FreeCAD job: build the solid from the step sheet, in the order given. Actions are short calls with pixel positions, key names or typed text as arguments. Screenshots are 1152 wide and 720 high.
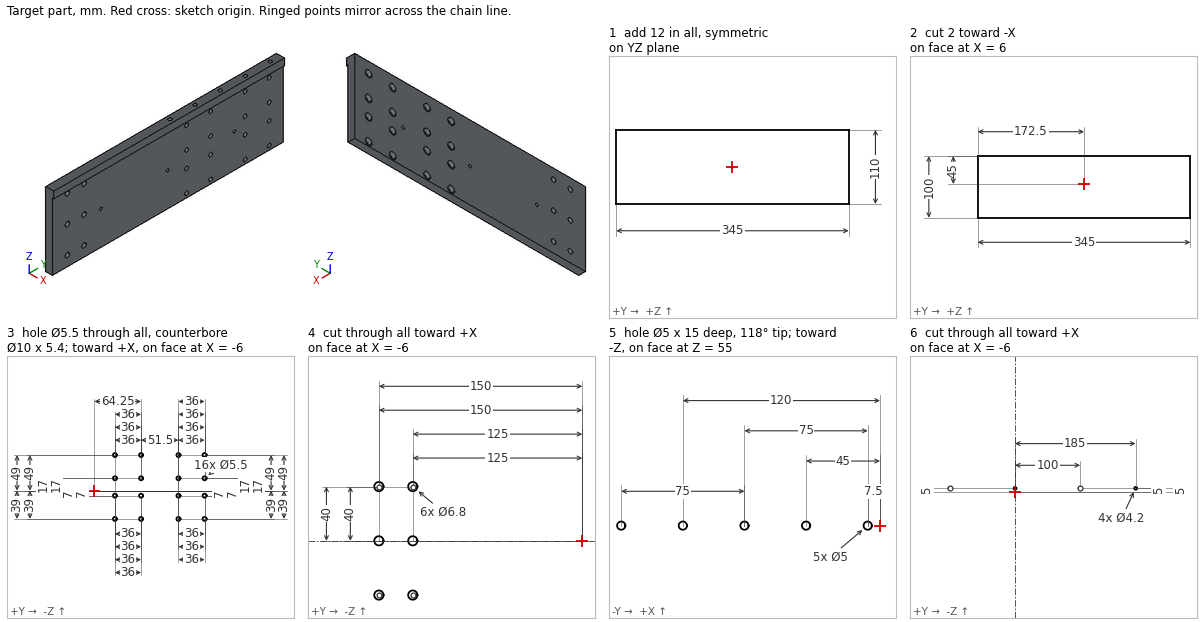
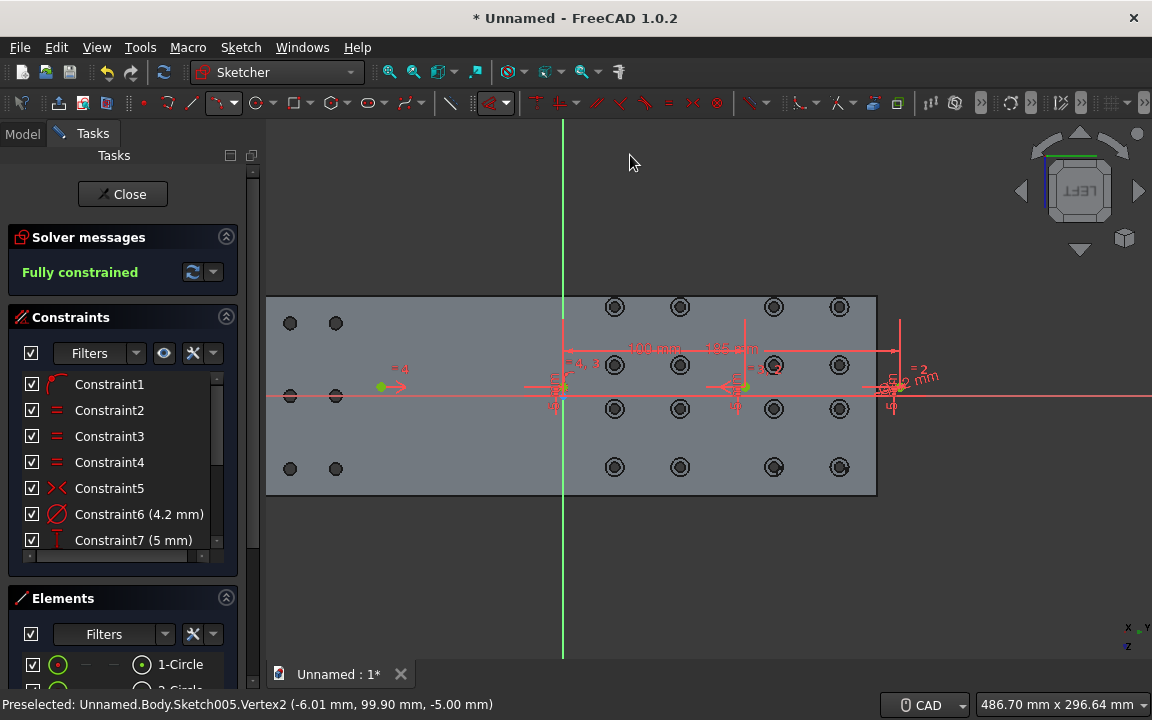
click(123, 194)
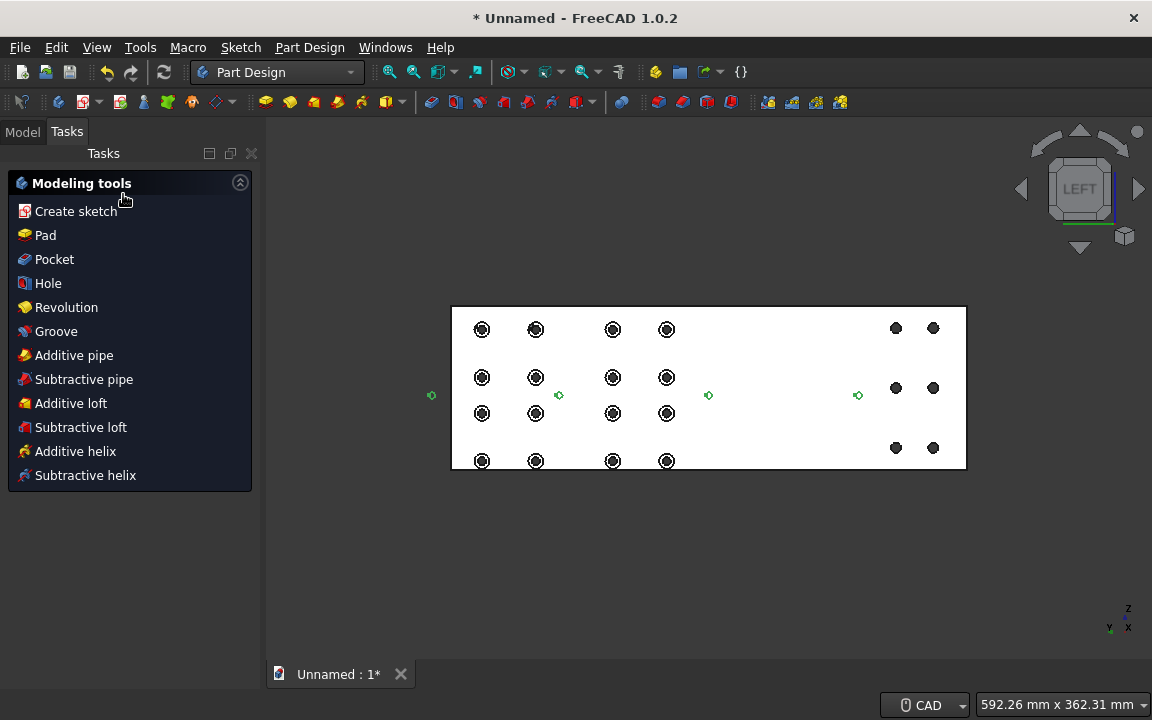
click(432, 102)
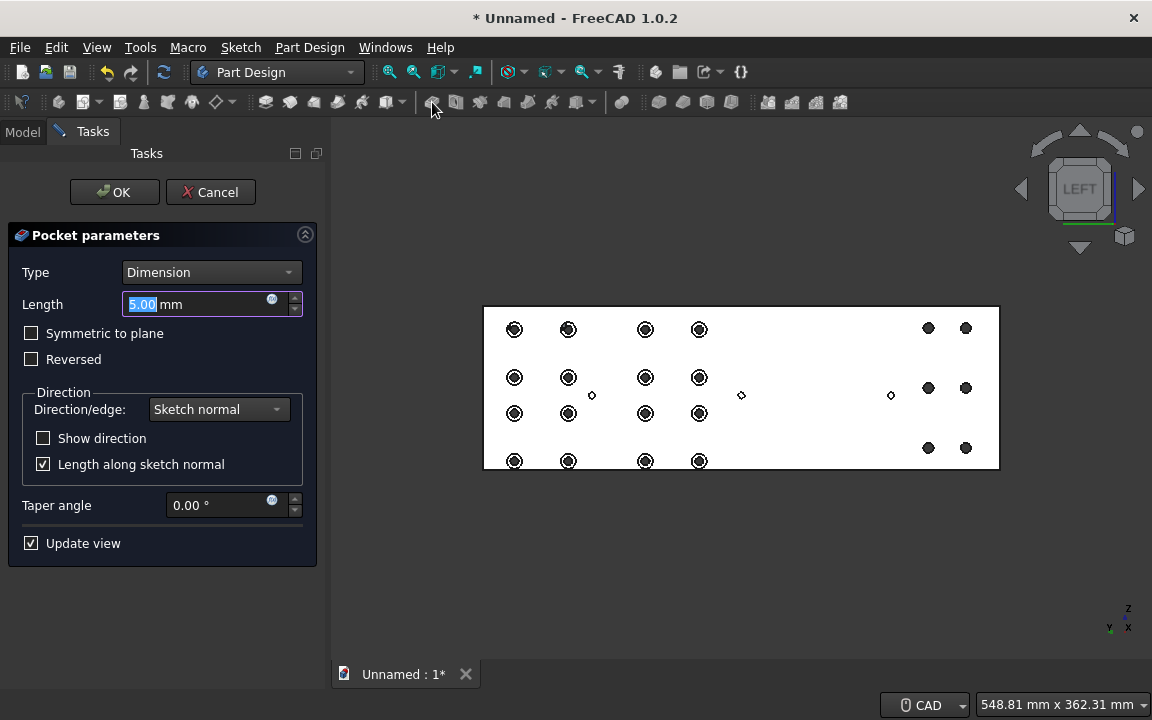
click(212, 272)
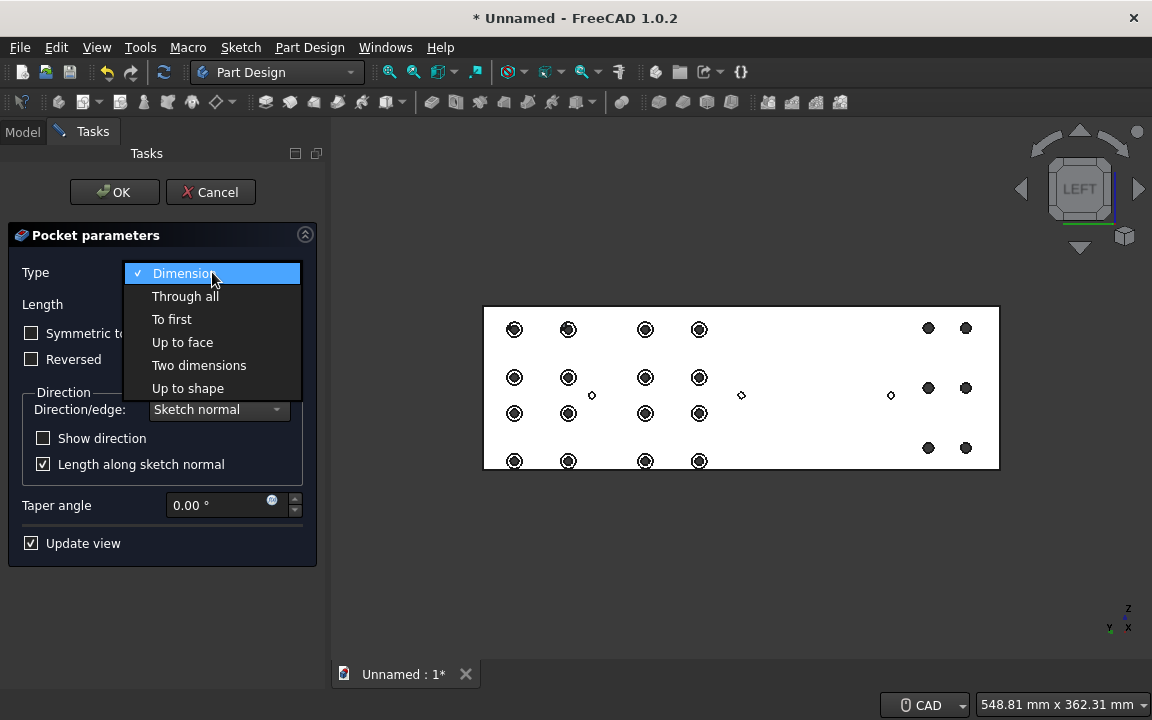
click(212, 296)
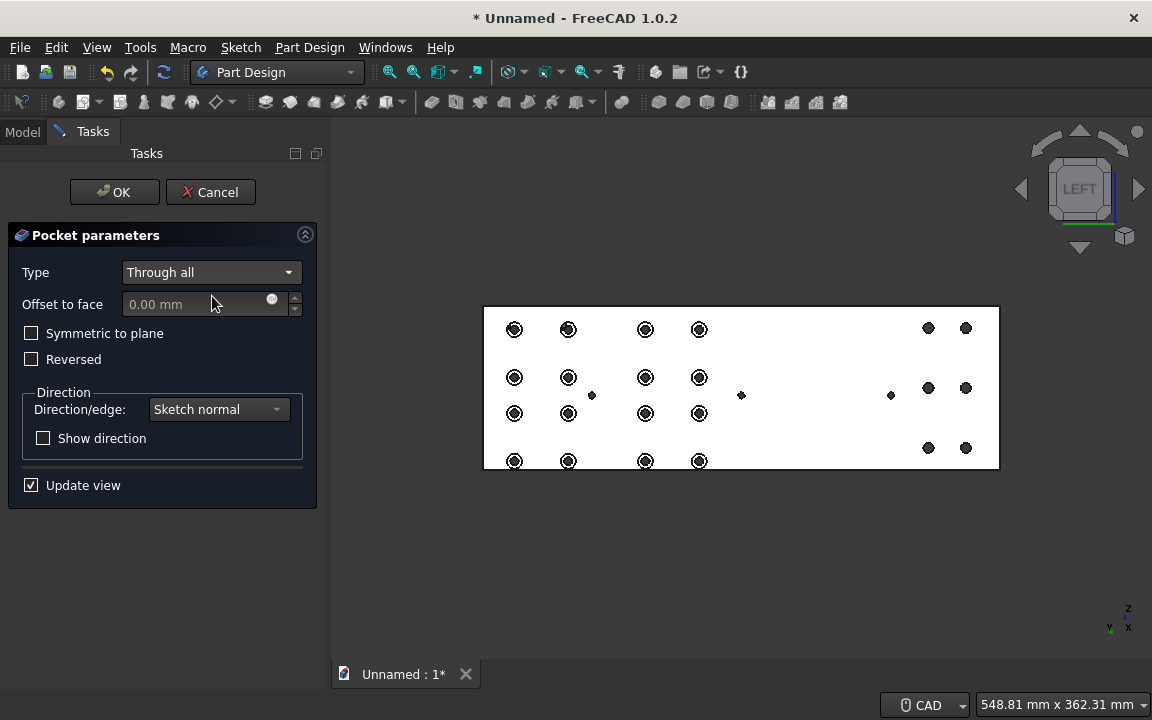
click(115, 192)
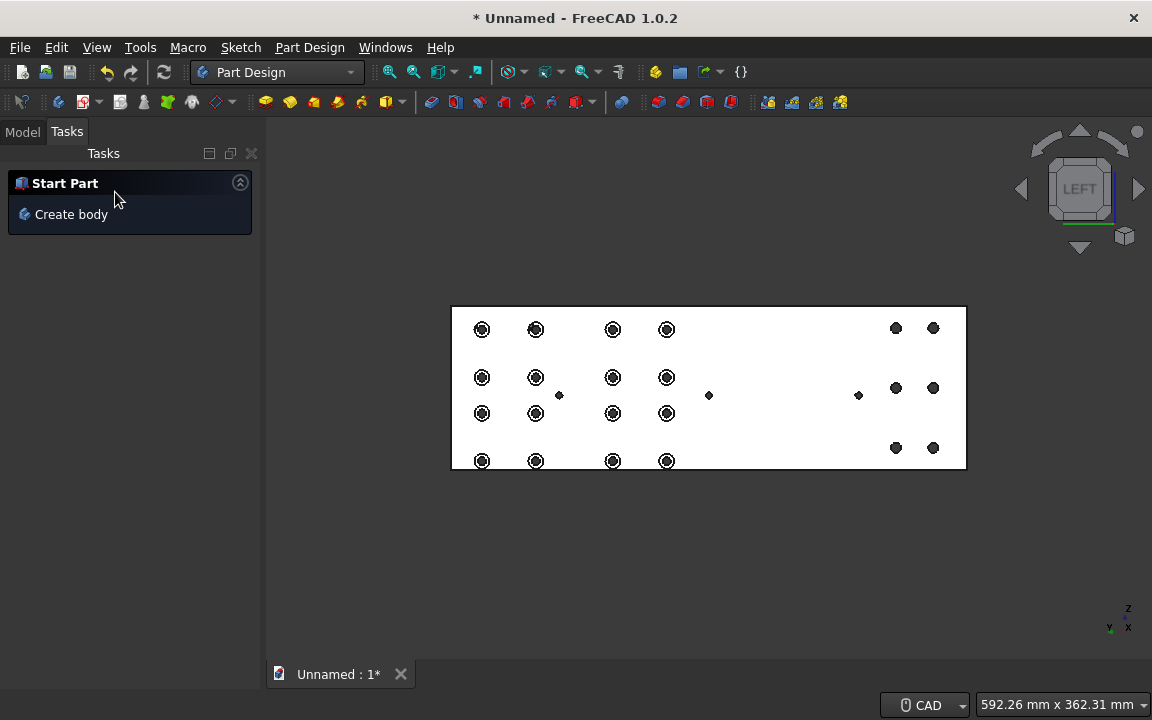
key(0)